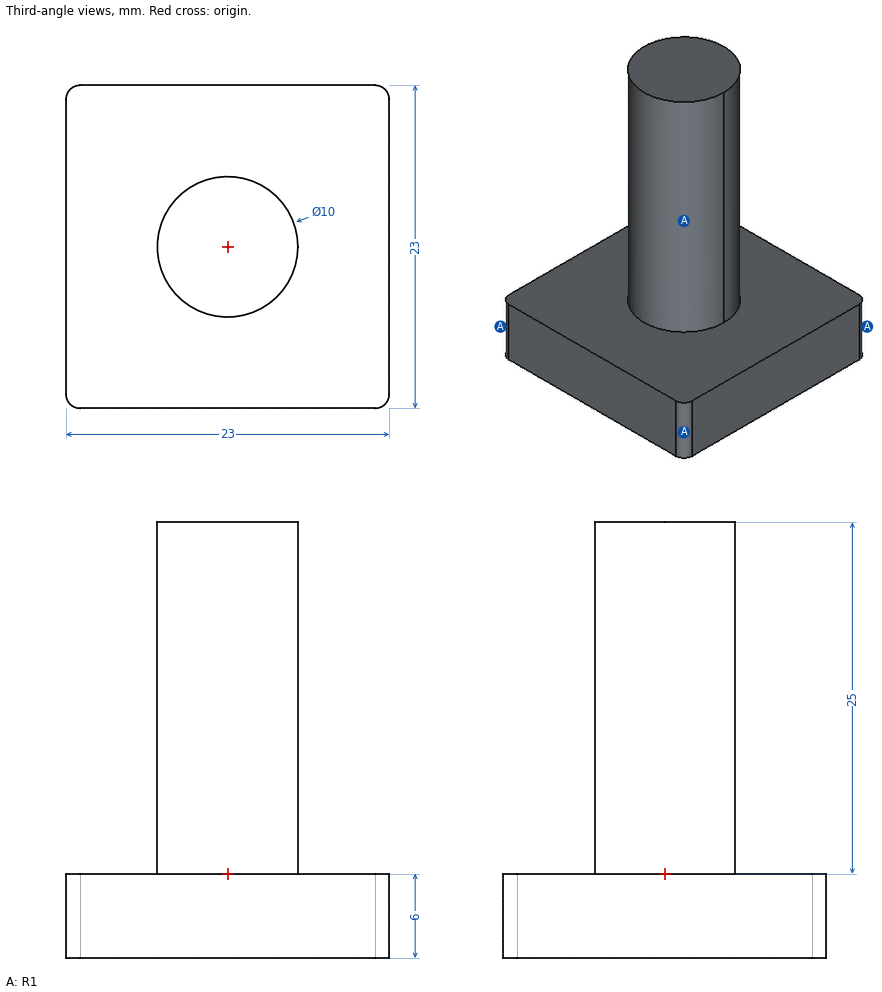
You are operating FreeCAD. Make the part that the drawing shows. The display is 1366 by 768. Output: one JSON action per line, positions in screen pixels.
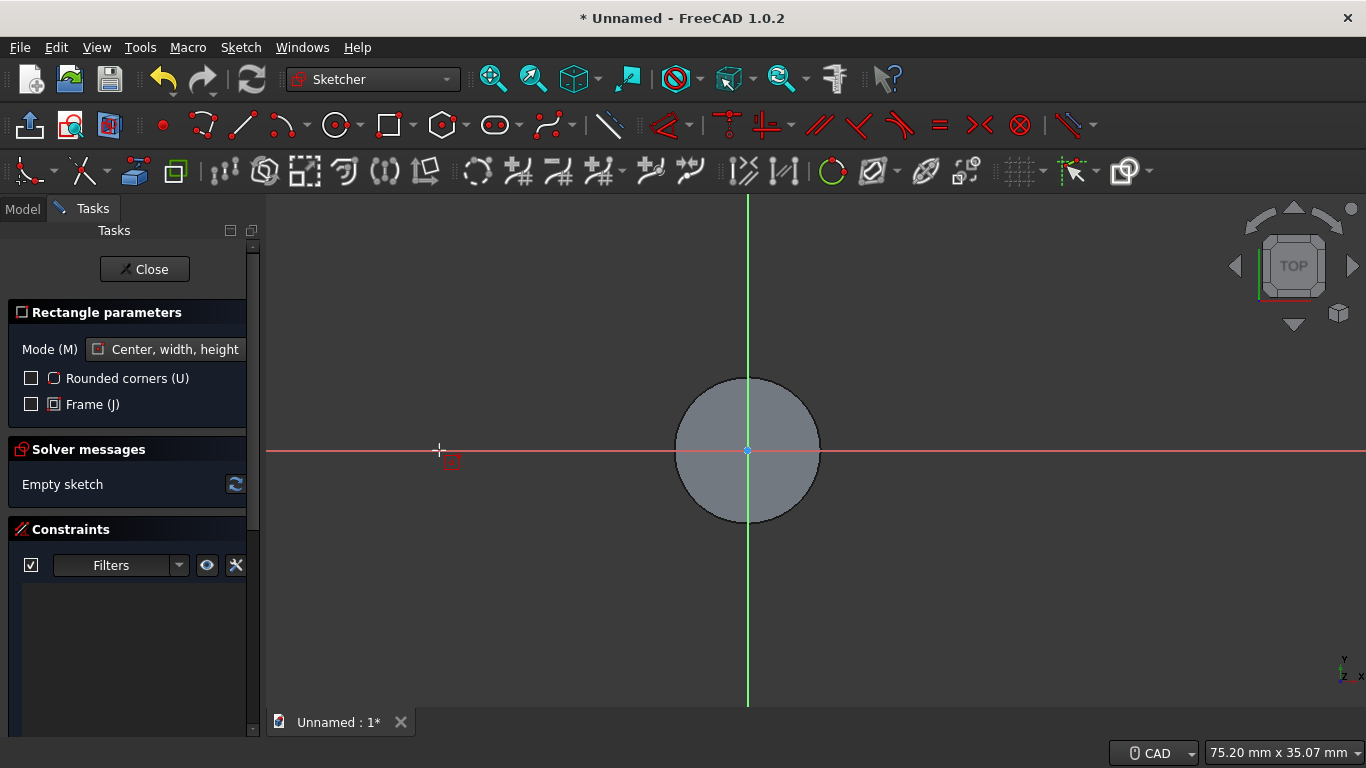
{"action": "left_click", "coordinate": [748, 450]}
{"action": "mouse_move", "coordinate": [916, 282]}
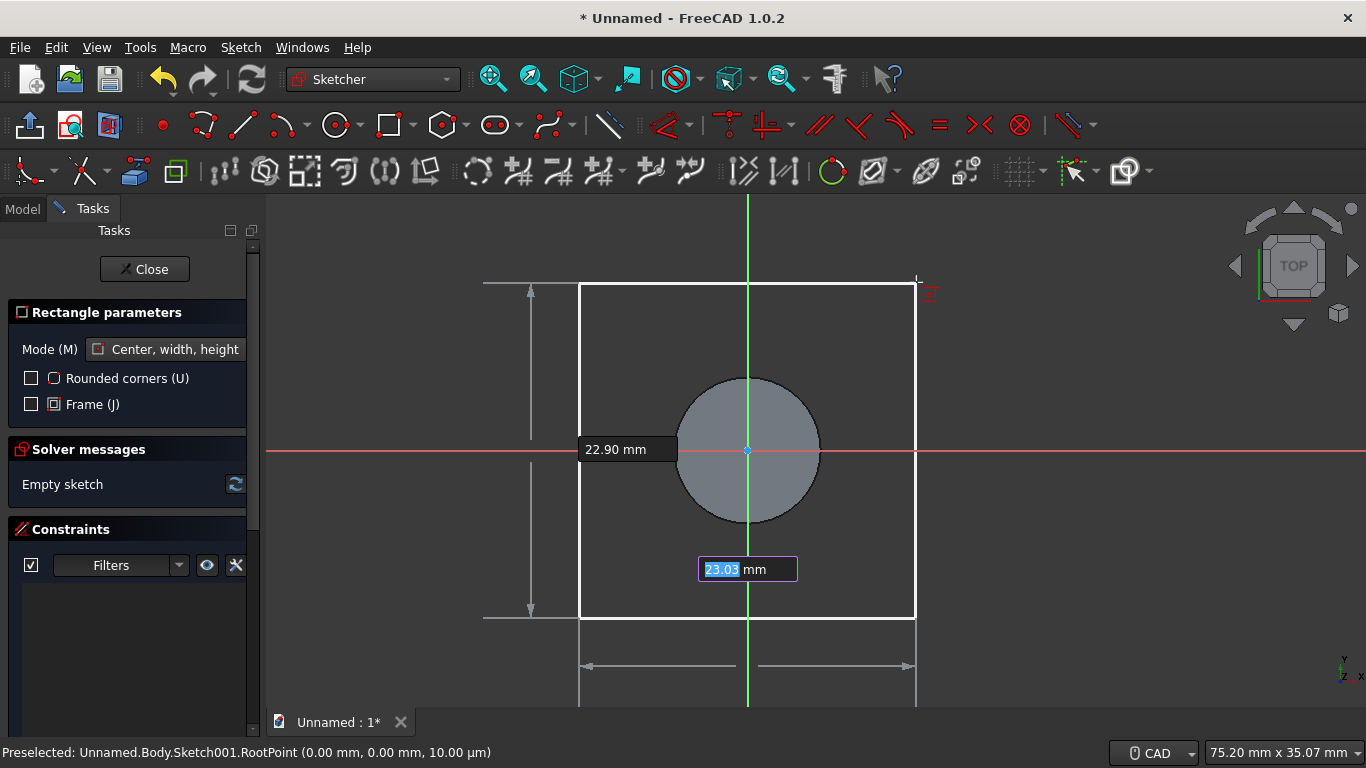
{"action": "type", "text": "23"}
{"action": "key", "text": "Tab"}
{"action": "type", "text": "23"}
{"action": "key", "text": "Return"}
{"action": "key", "text": "Escape"}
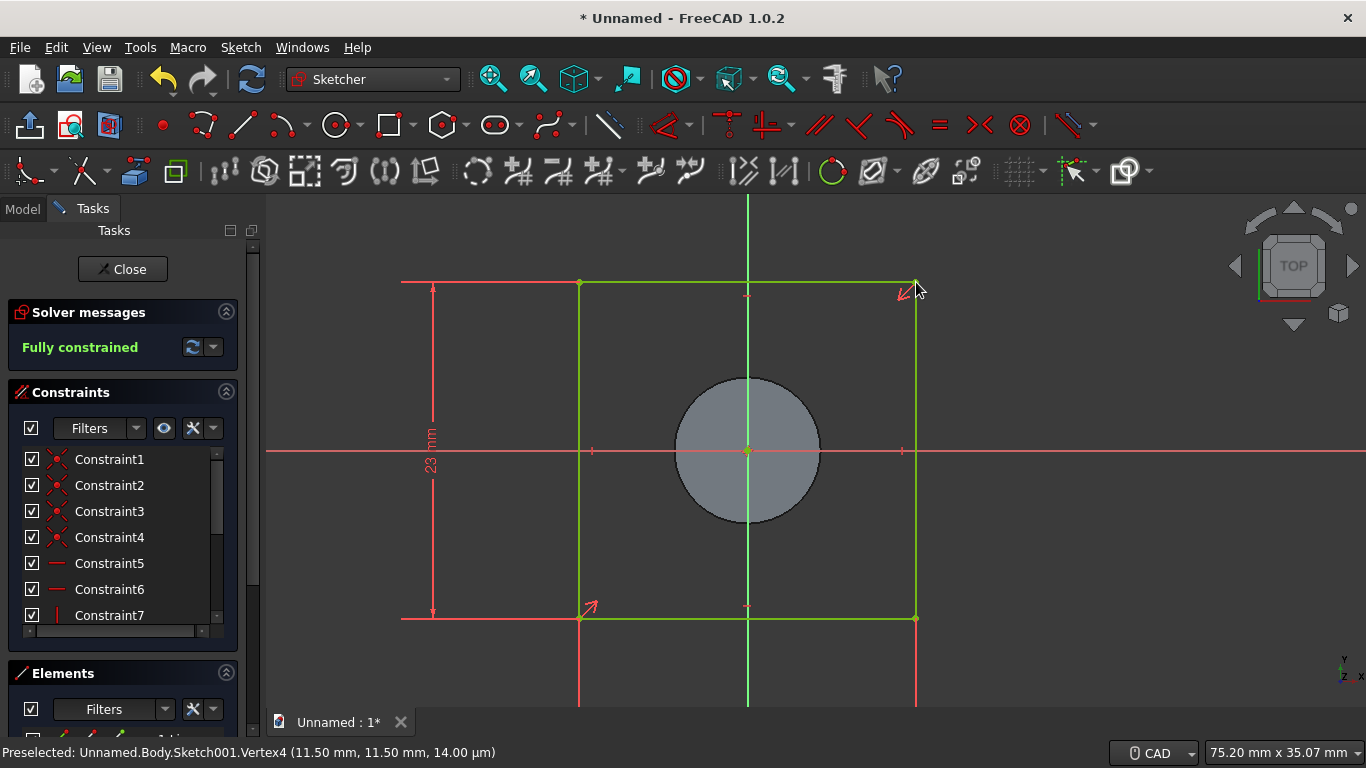
{"action": "left_click", "coordinate": [123, 269]}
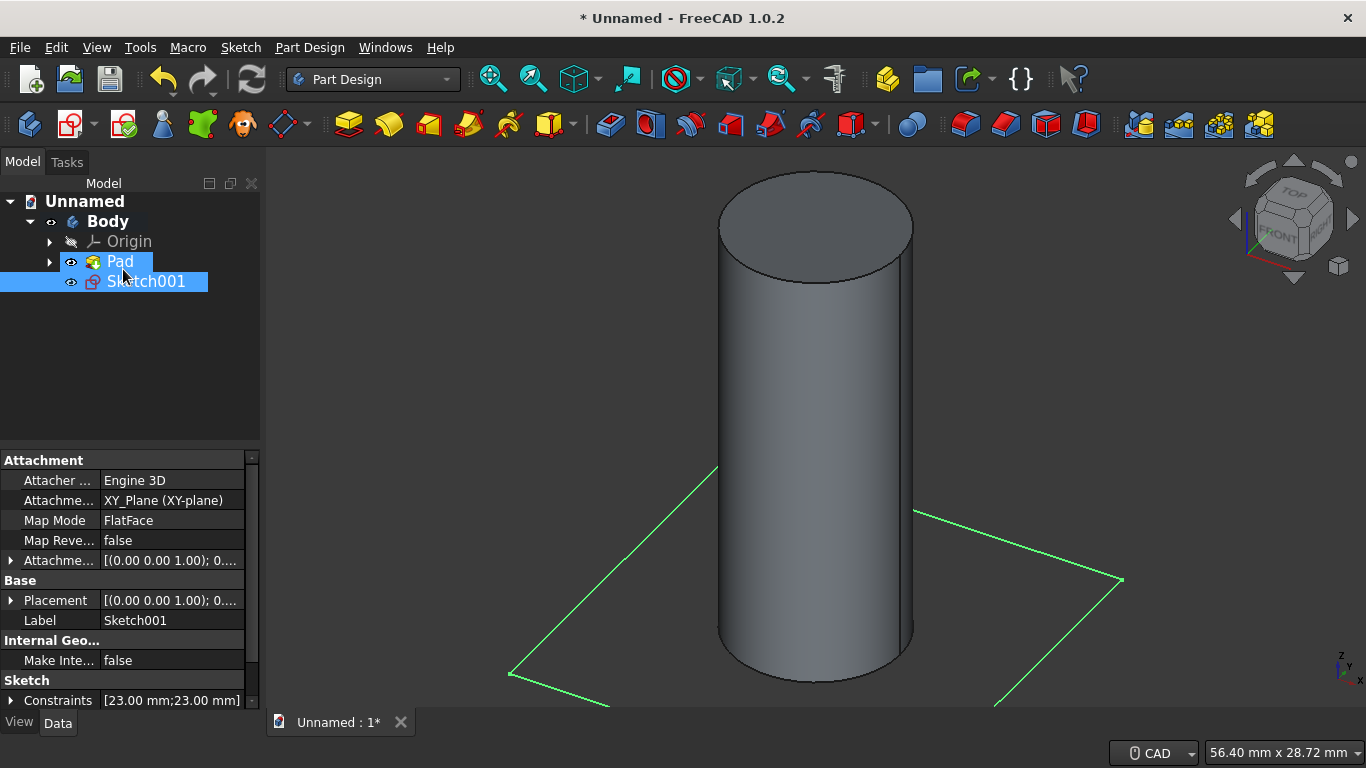
{"action": "left_click", "coordinate": [350, 124]}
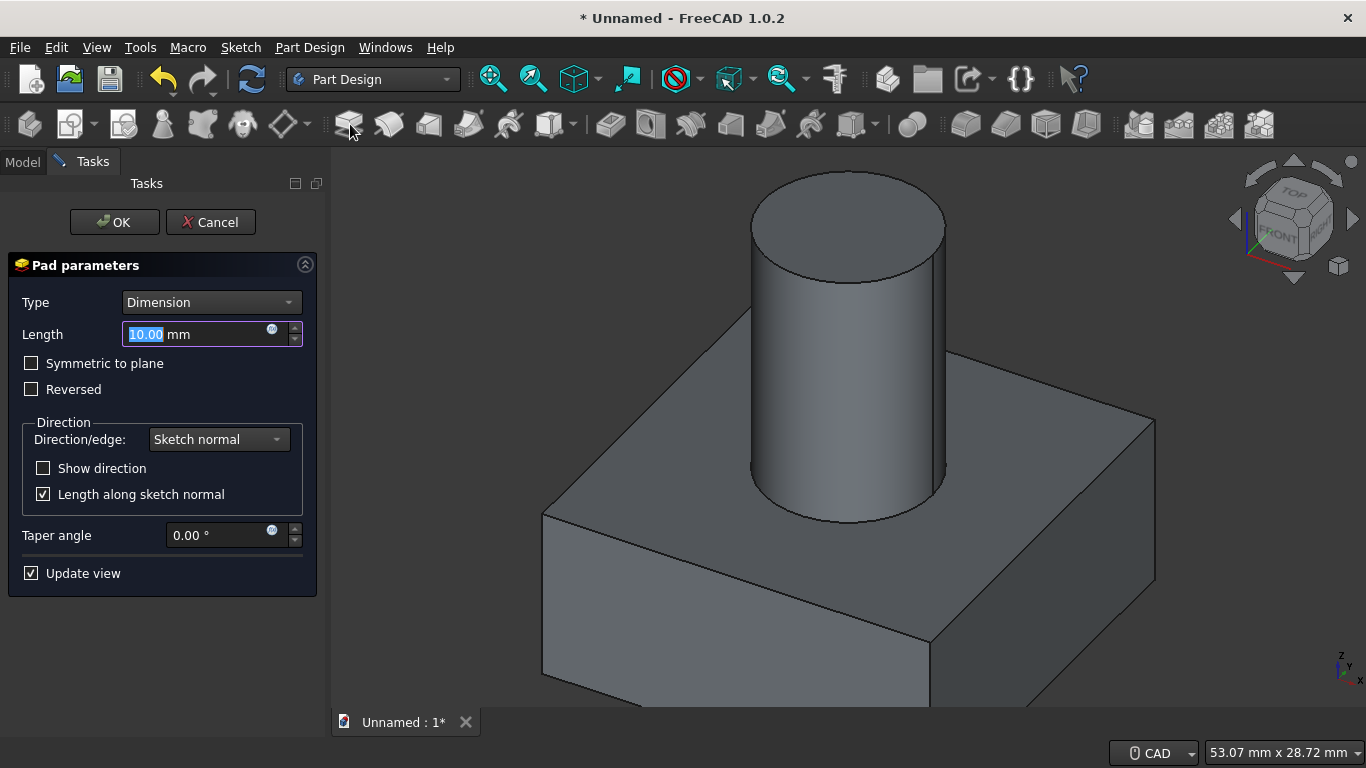
{"action": "type", "text": "6"}
{"action": "key", "text": "Tab"}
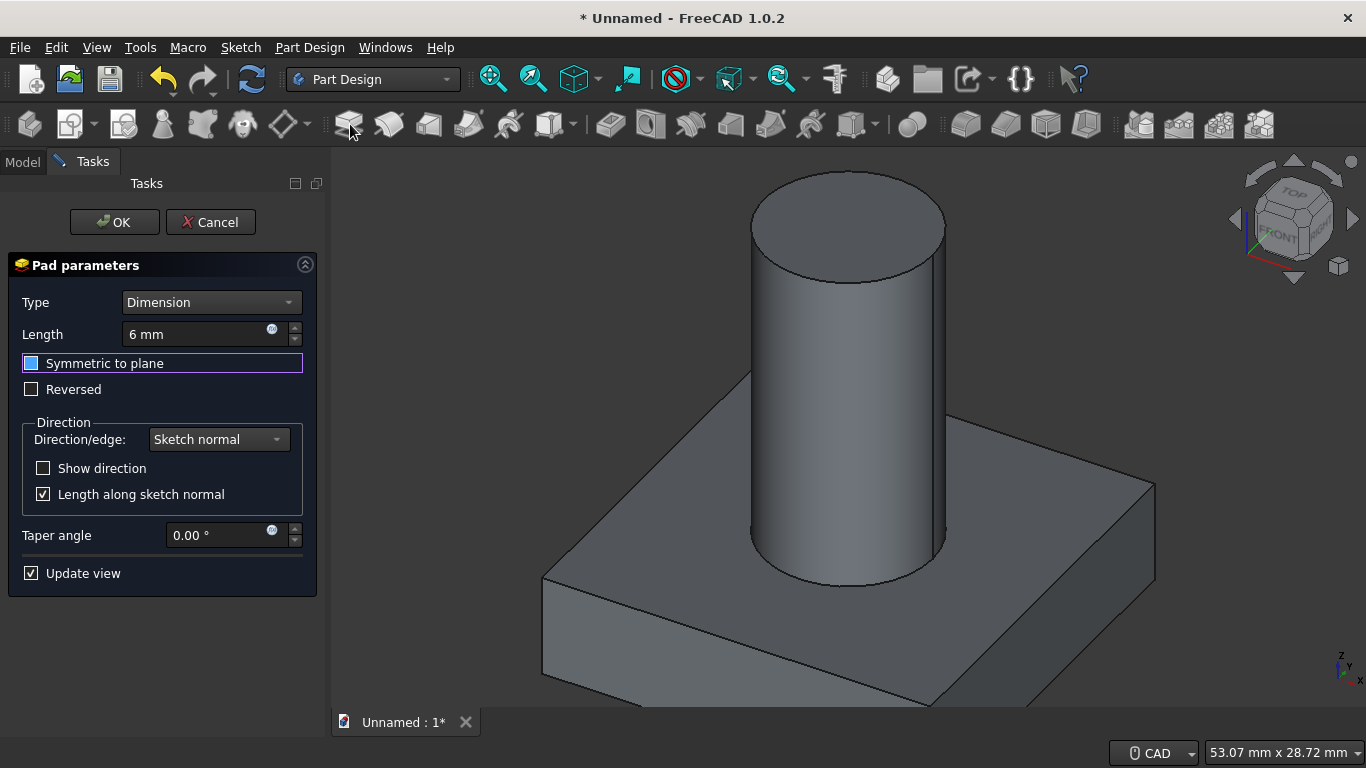
{"action": "left_click", "coordinate": [30, 389]}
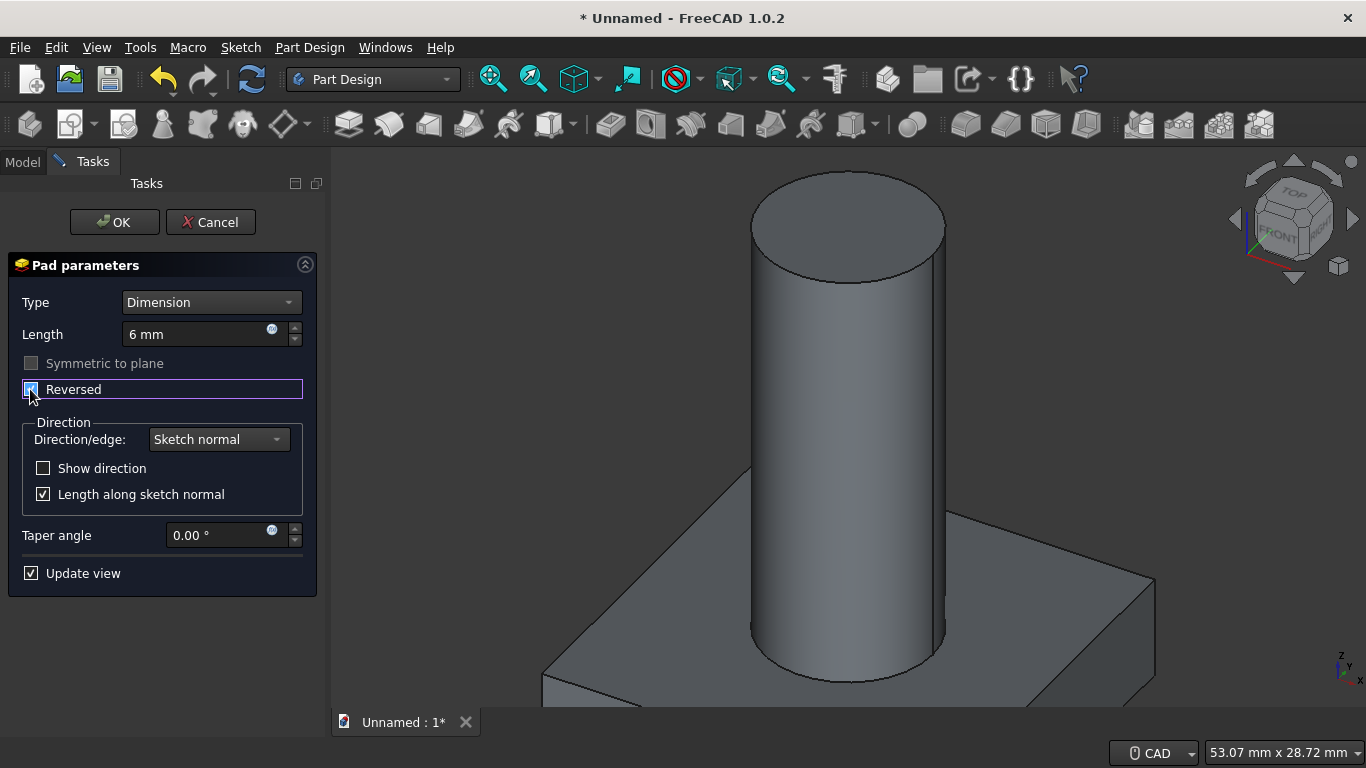
{"action": "left_click", "coordinate": [115, 222]}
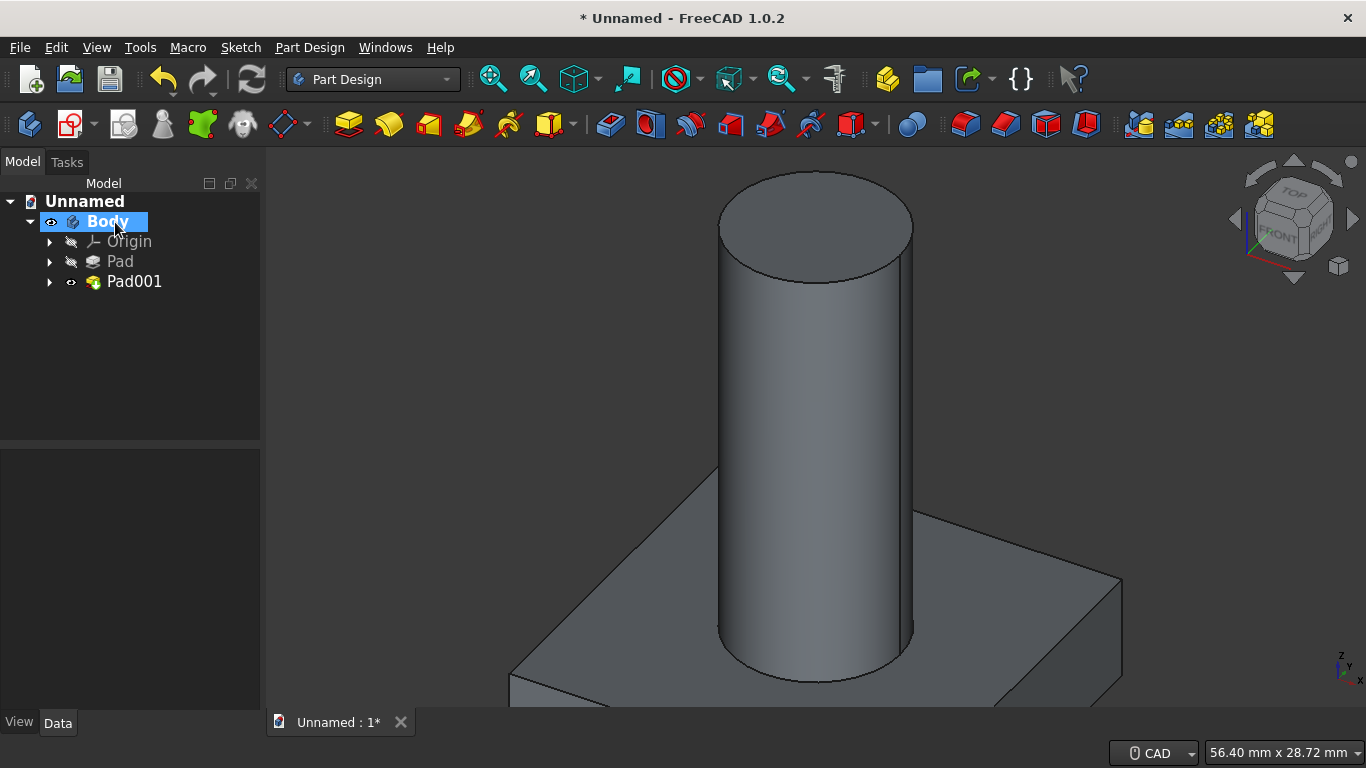
{"action": "key", "text": "v f"}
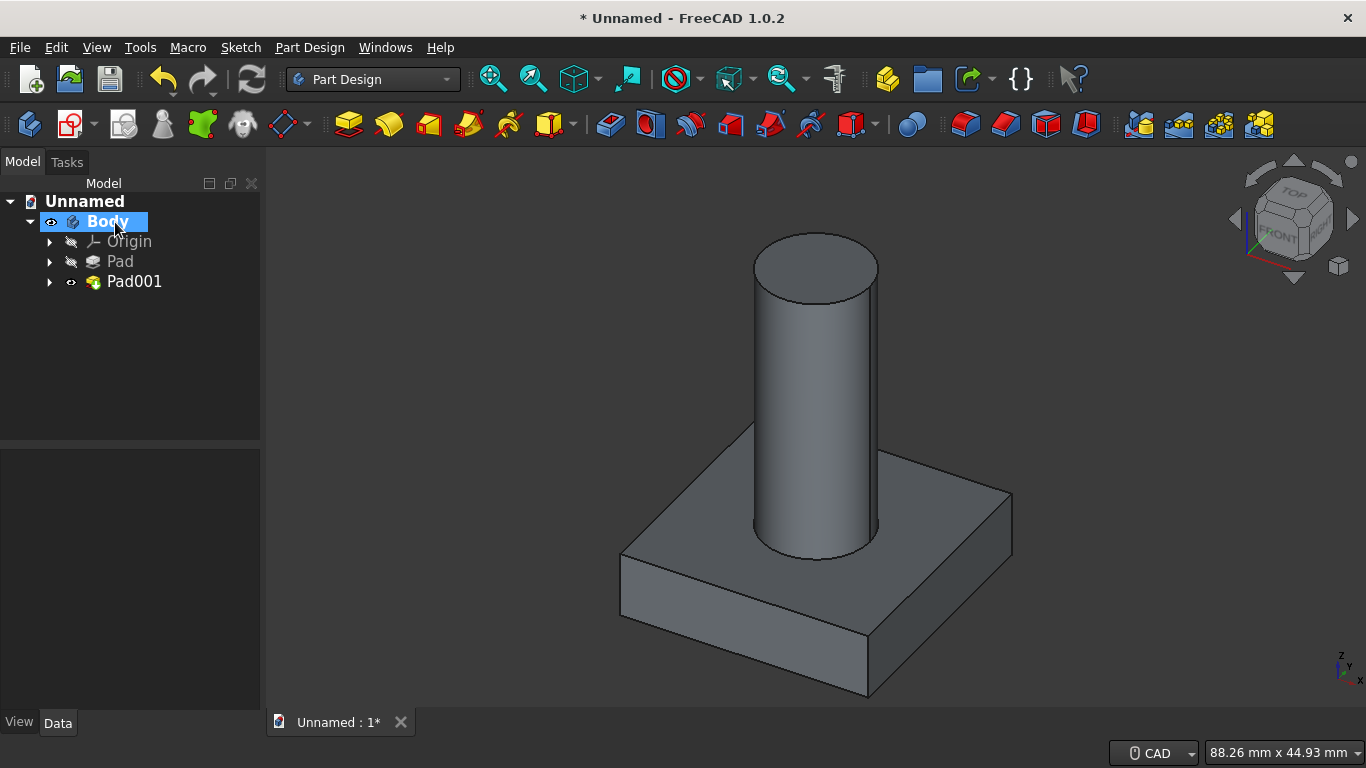
{"action": "left_click", "coordinate": [868, 666]}